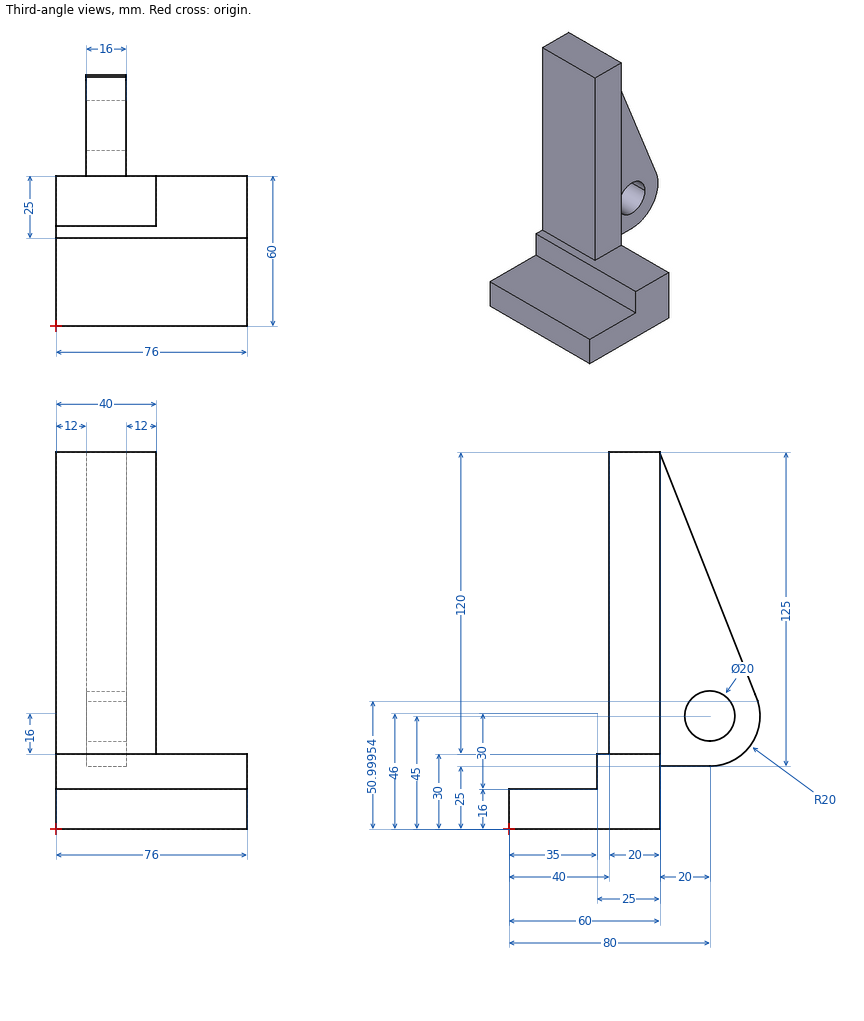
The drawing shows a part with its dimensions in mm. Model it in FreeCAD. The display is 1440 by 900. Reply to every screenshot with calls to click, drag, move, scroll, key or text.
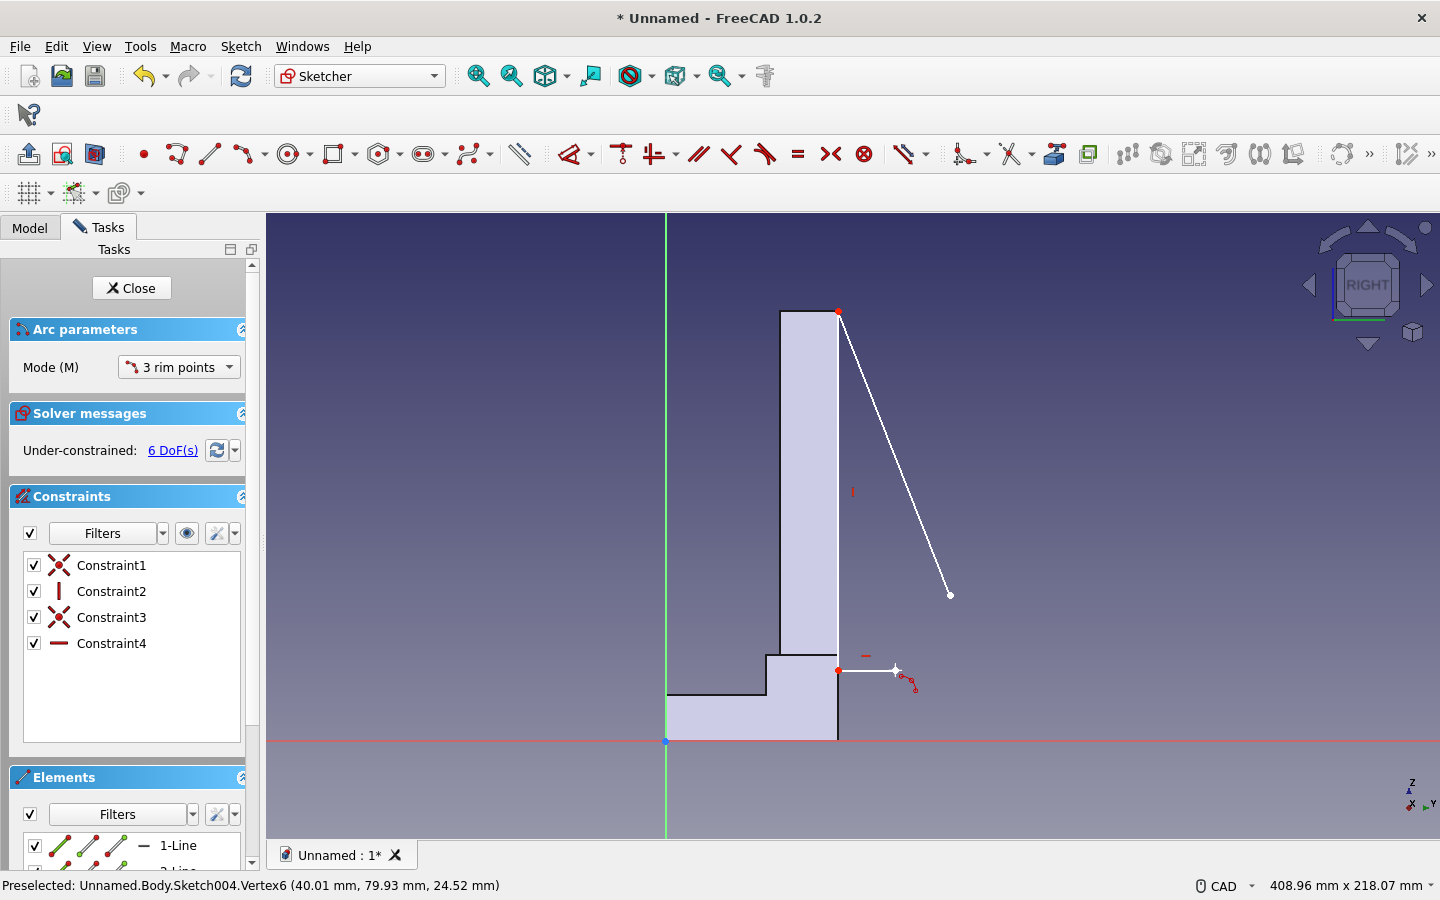
click(895, 671)
click(950, 596)
click(941, 646)
key(Escape)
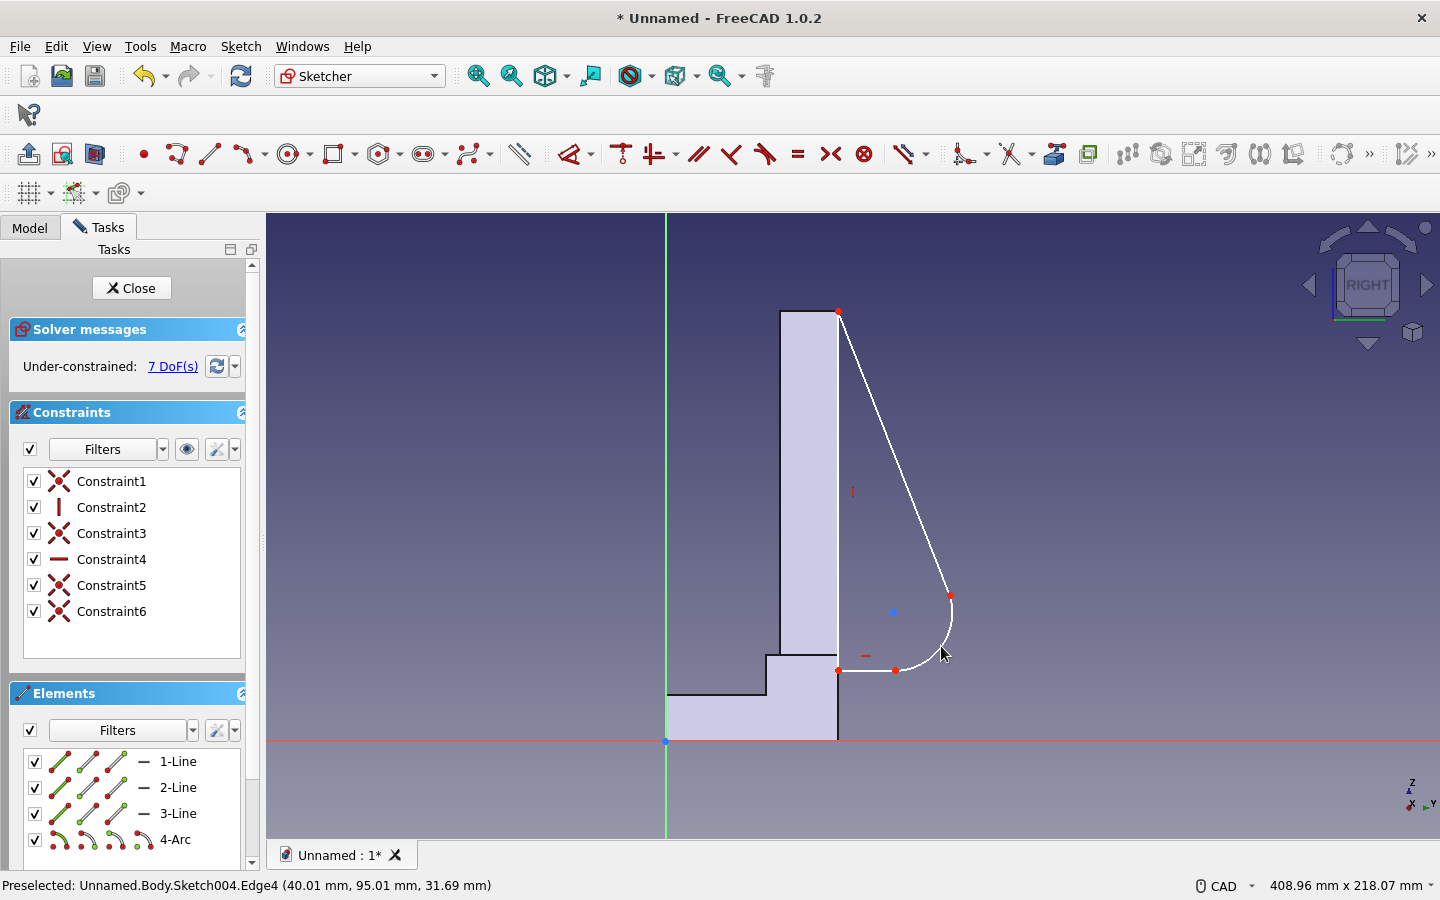
click(855, 671)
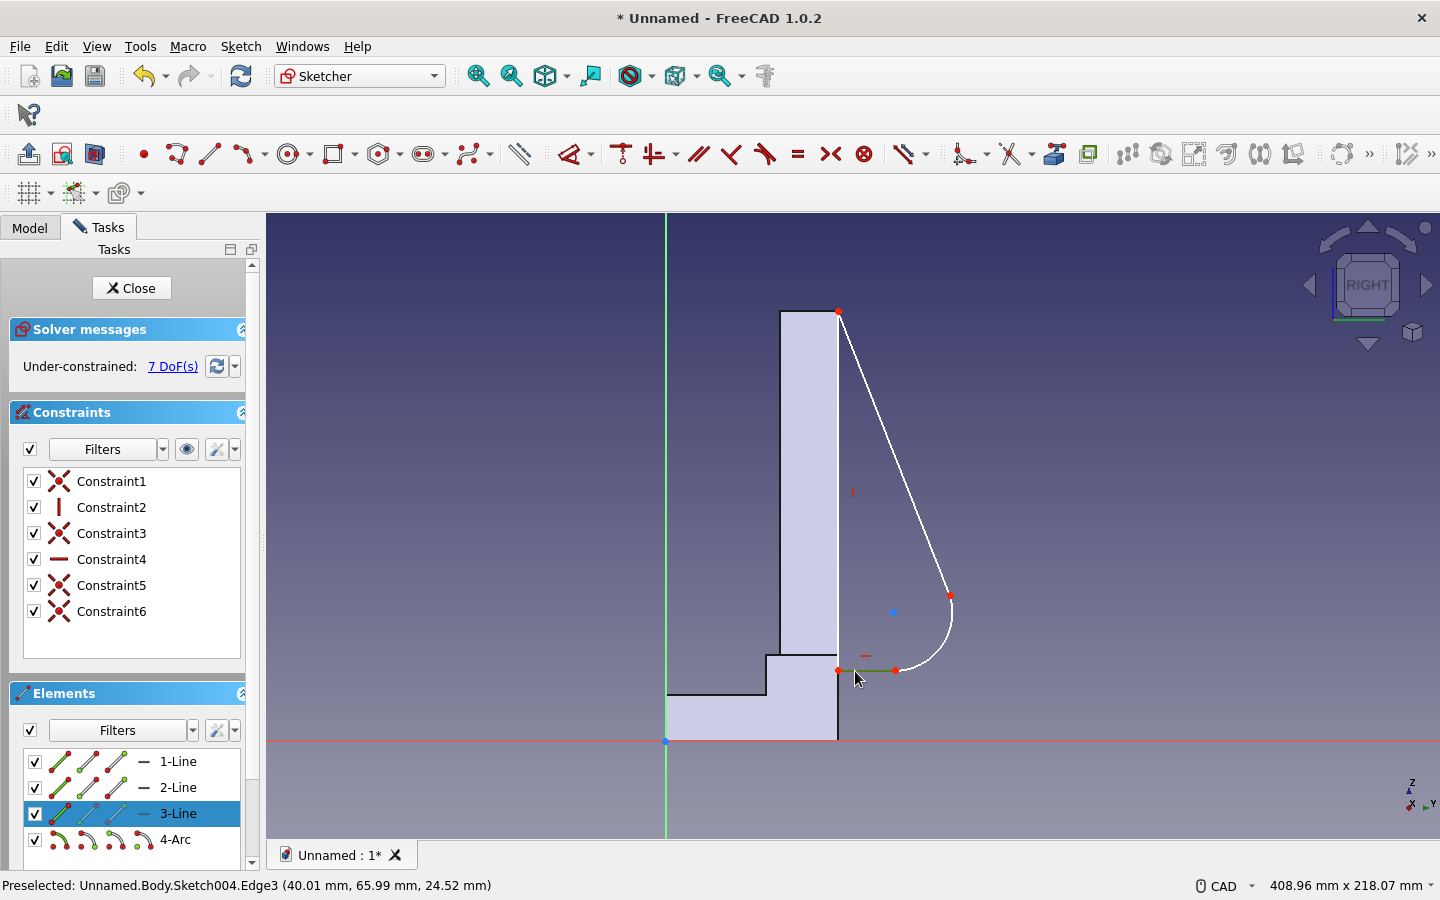
click(925, 662)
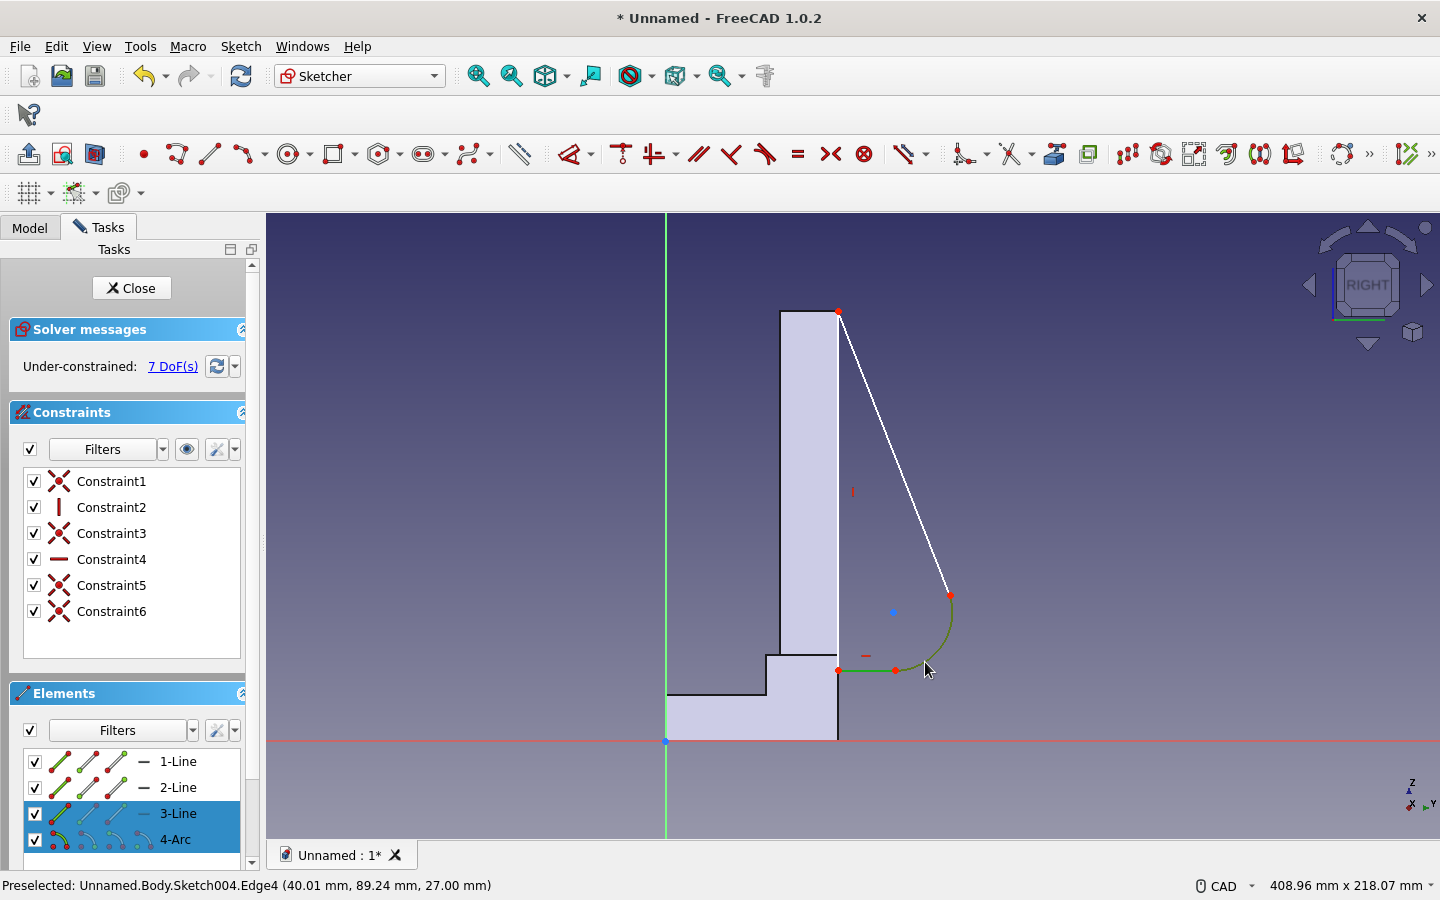
click(765, 154)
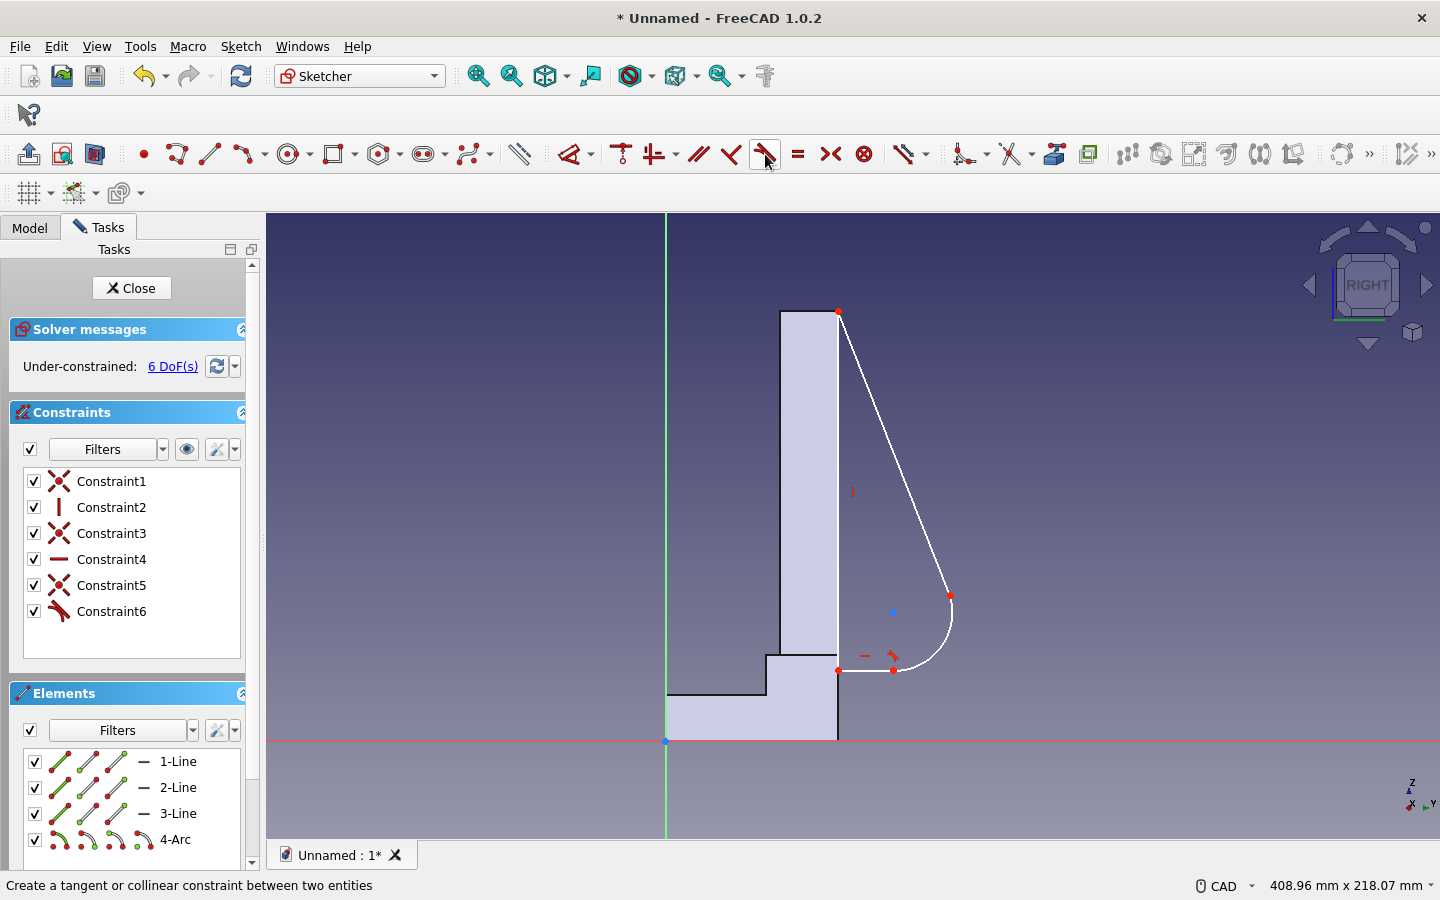
click(568, 154)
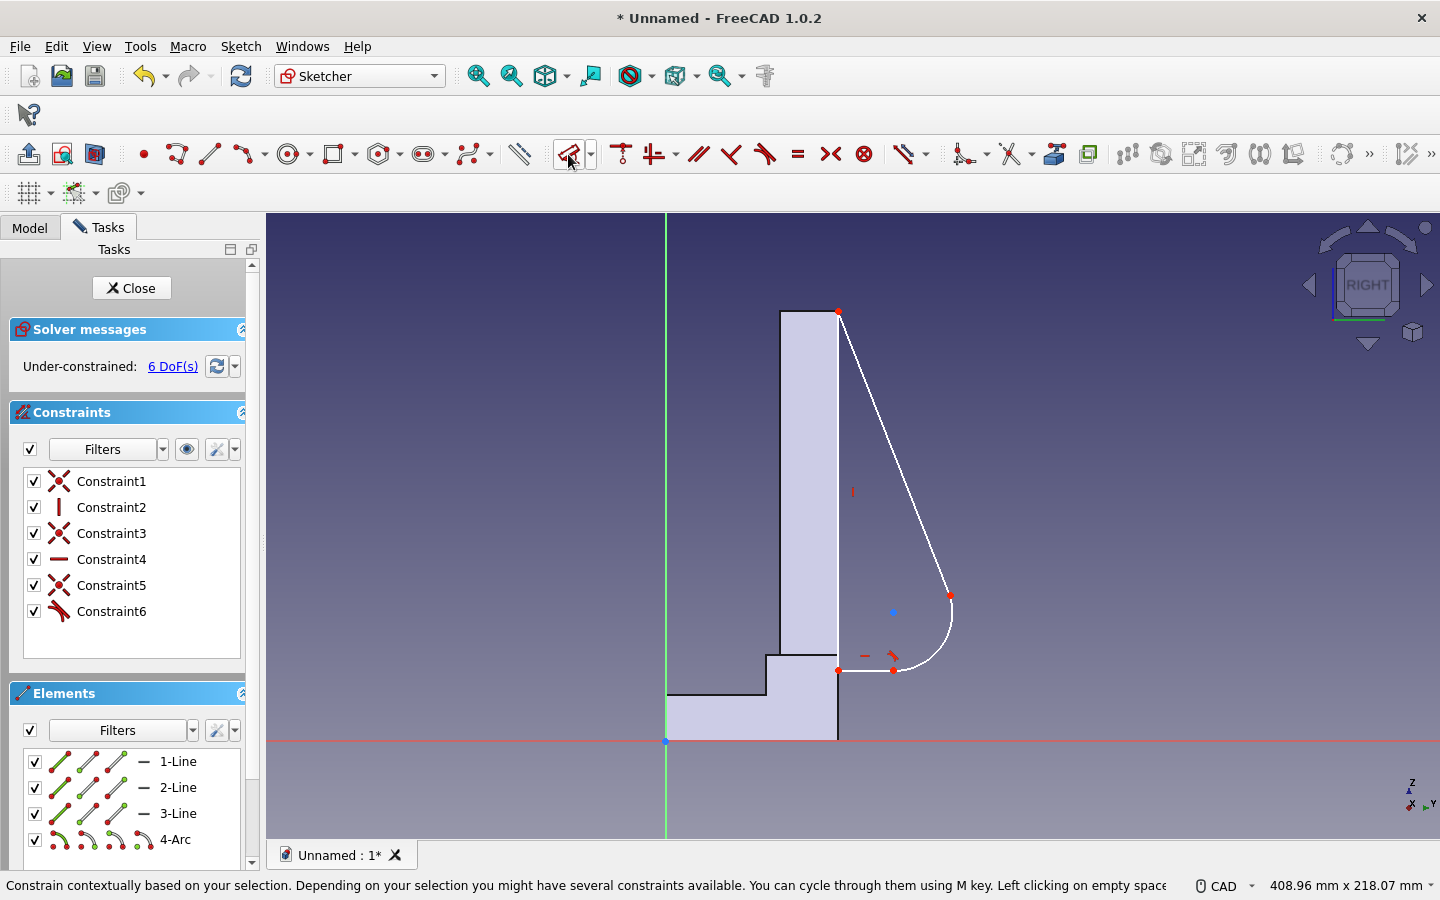
click(925, 662)
click(942, 689)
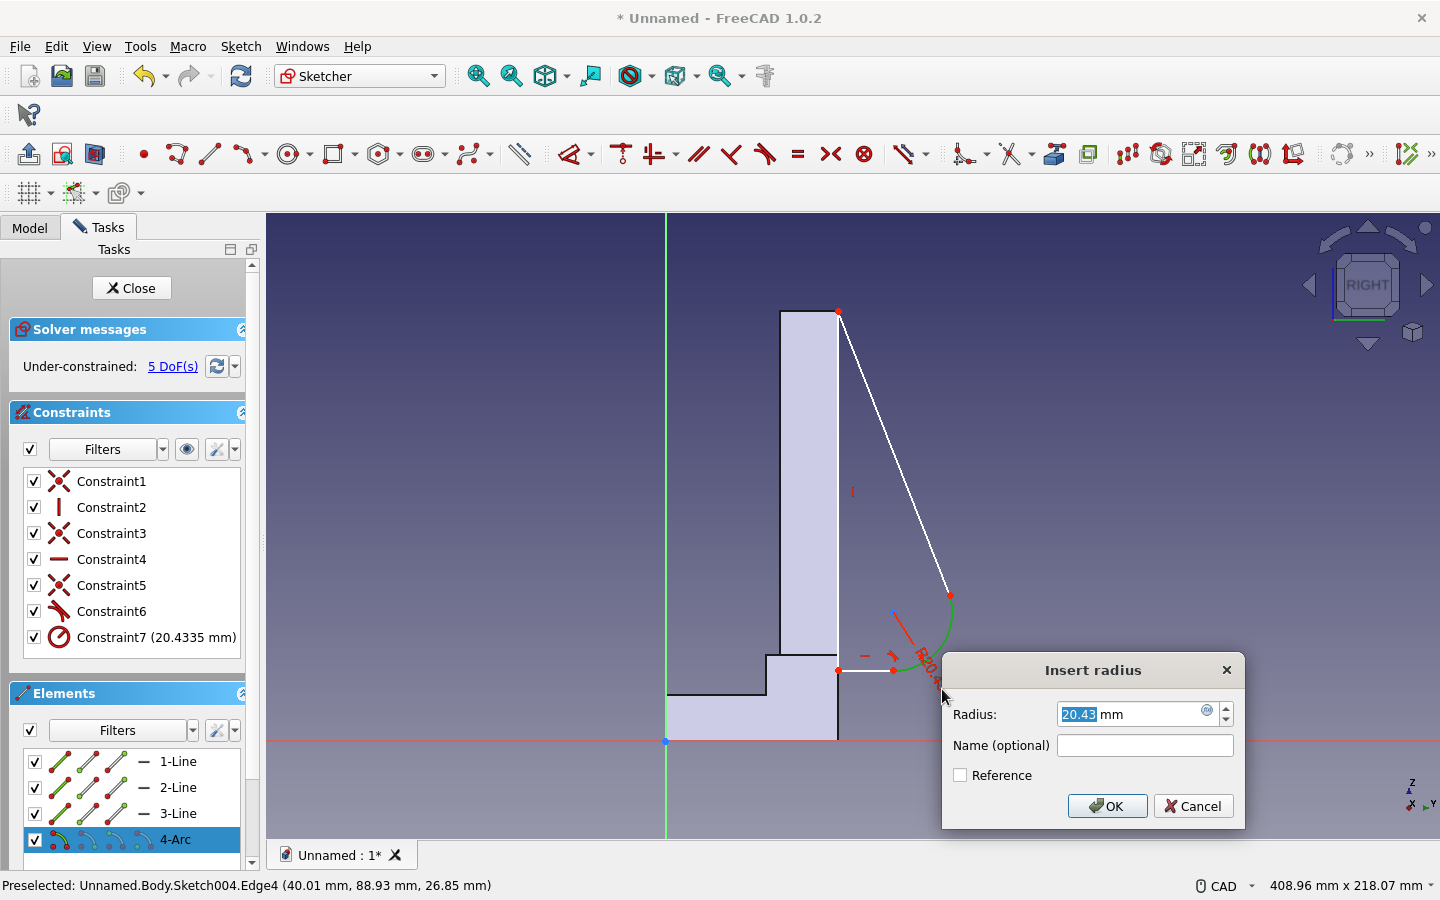
text(20)
key(Return)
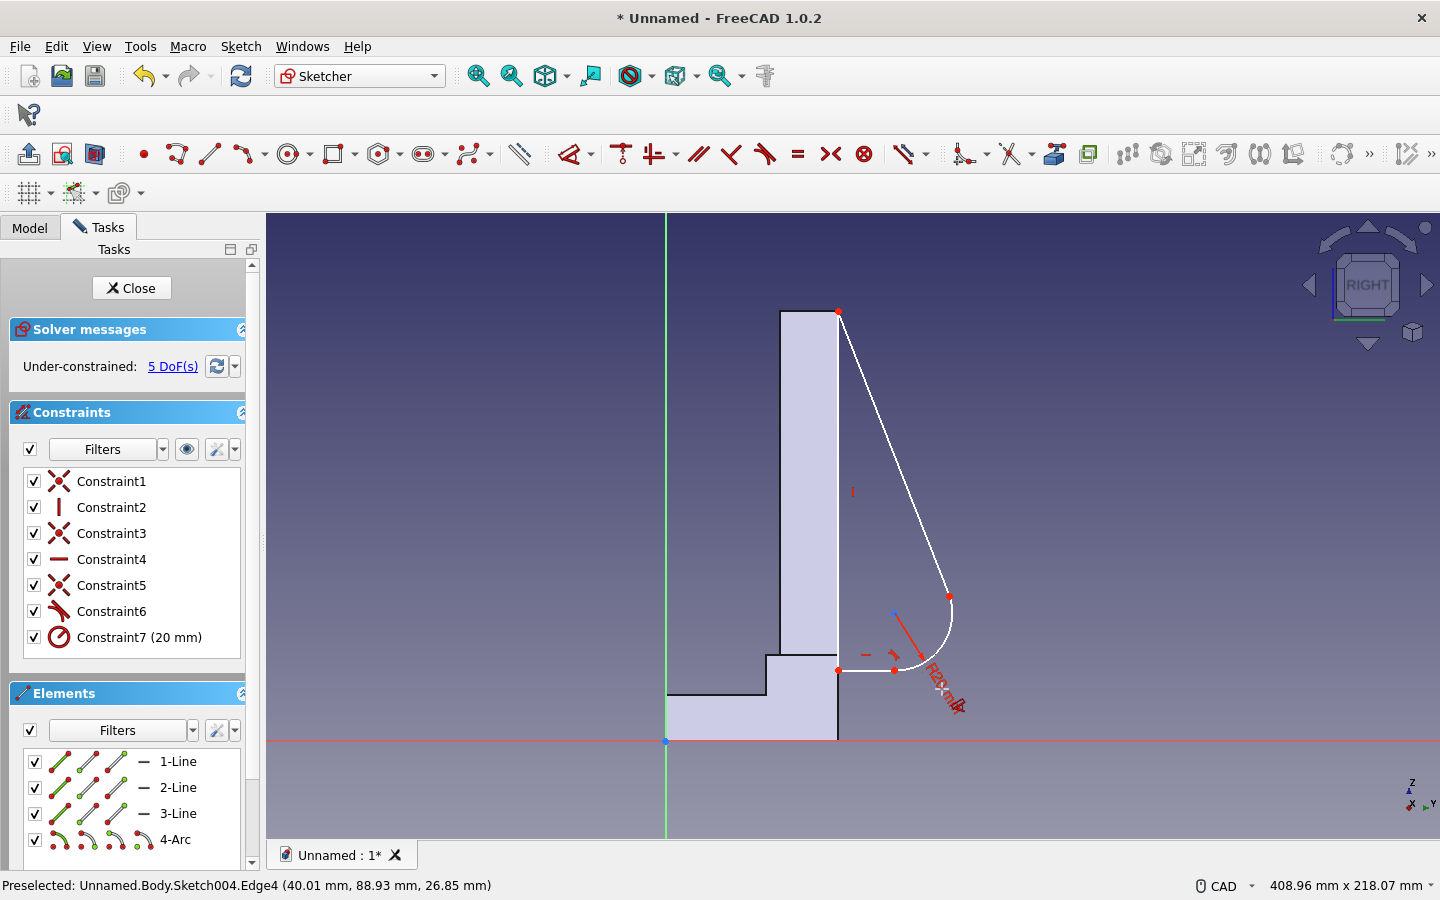
click(855, 671)
click(866, 705)